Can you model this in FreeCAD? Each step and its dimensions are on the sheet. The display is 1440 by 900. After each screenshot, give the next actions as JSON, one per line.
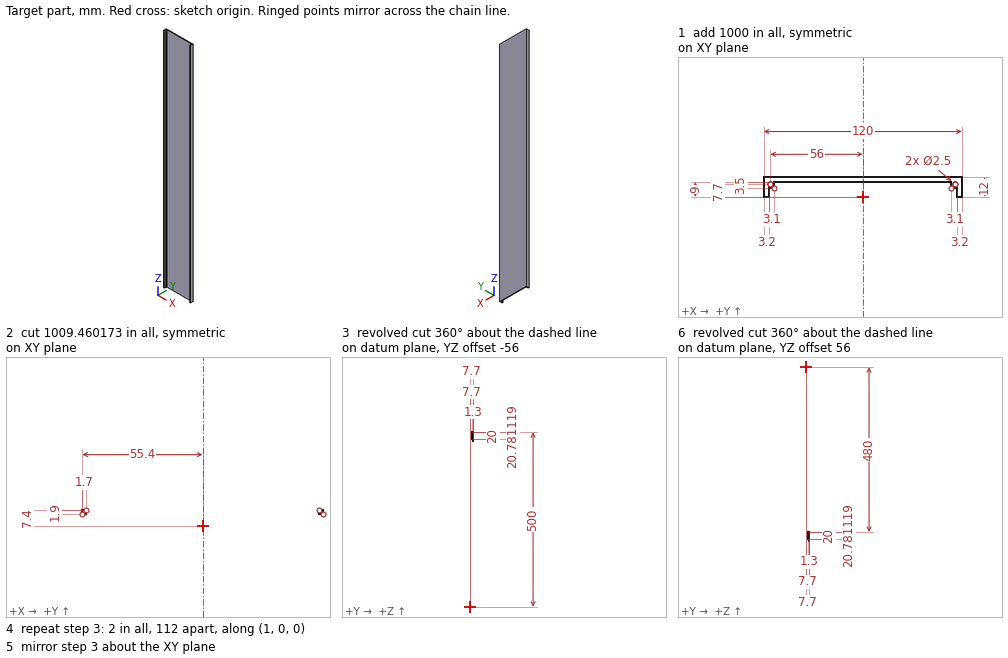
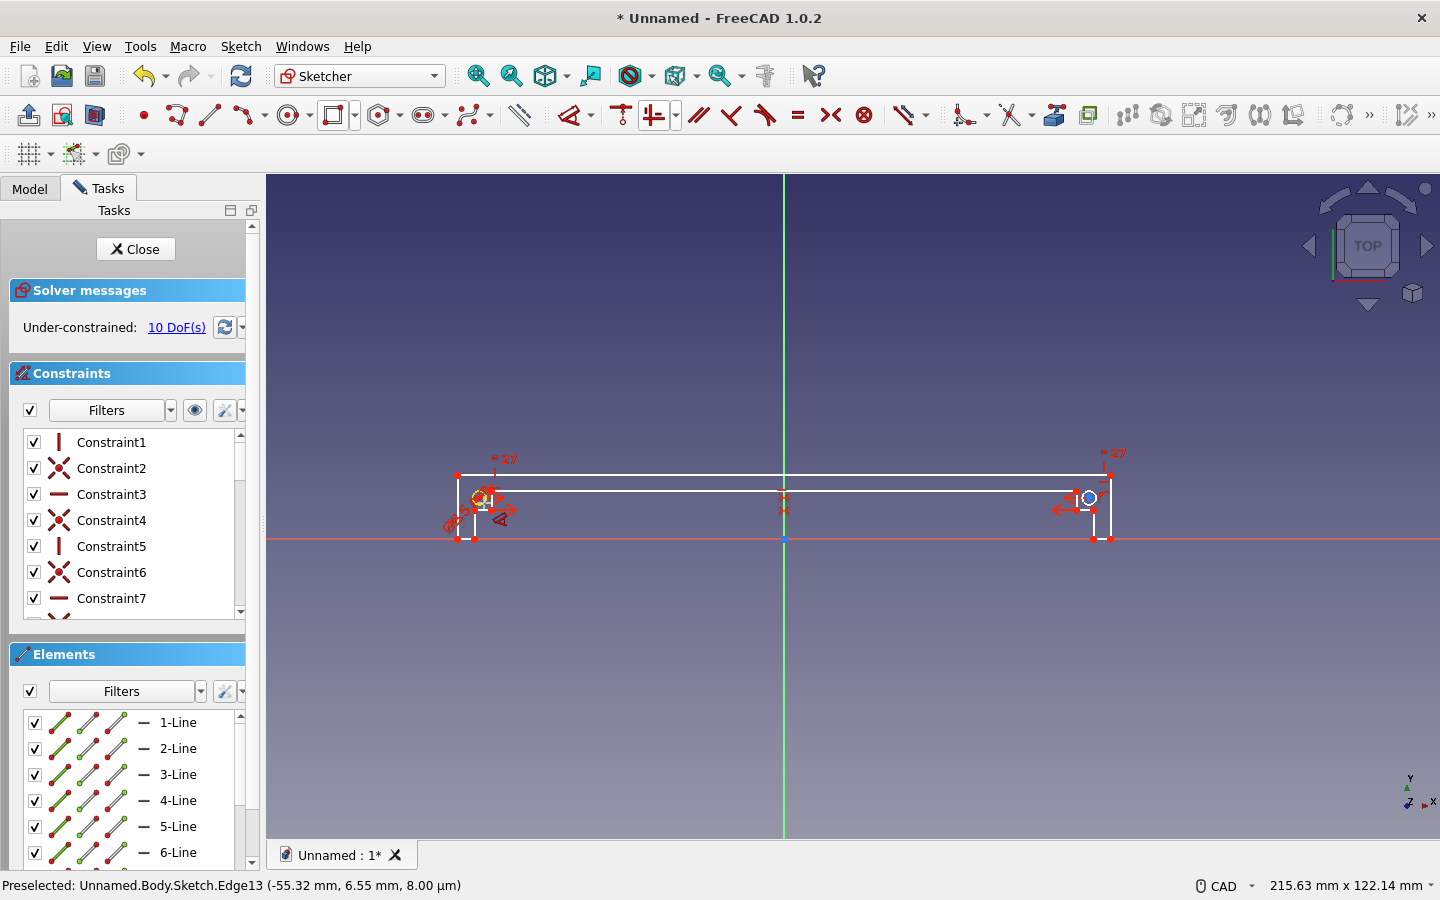
{"action": "left_click", "coordinate": [1111, 520]}
{"action": "left_click", "coordinate": [1145, 507]}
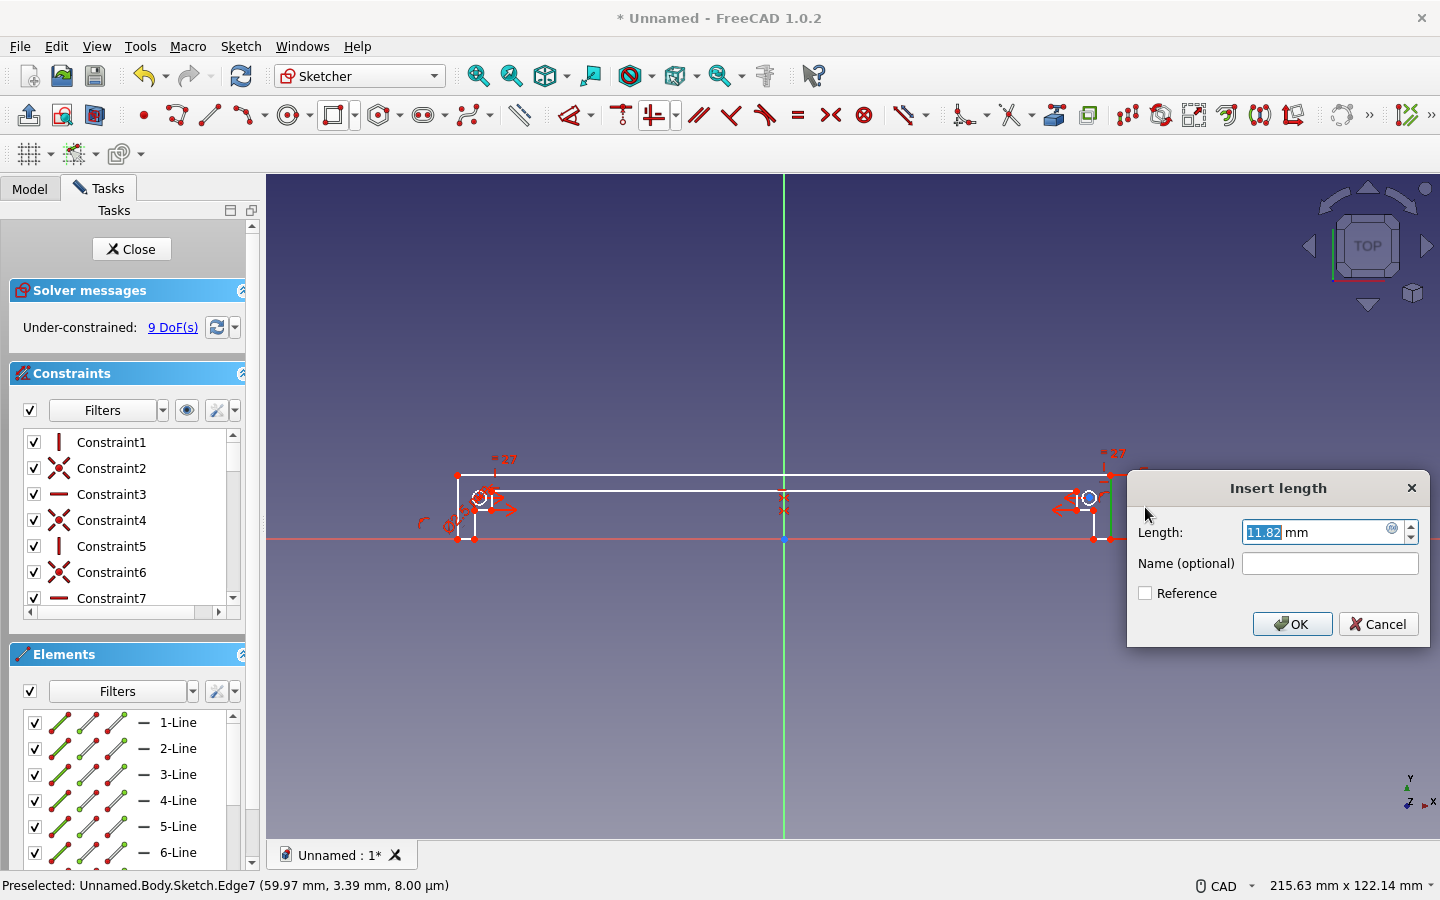
{"action": "type", "text": "12"}
{"action": "key", "text": "Return"}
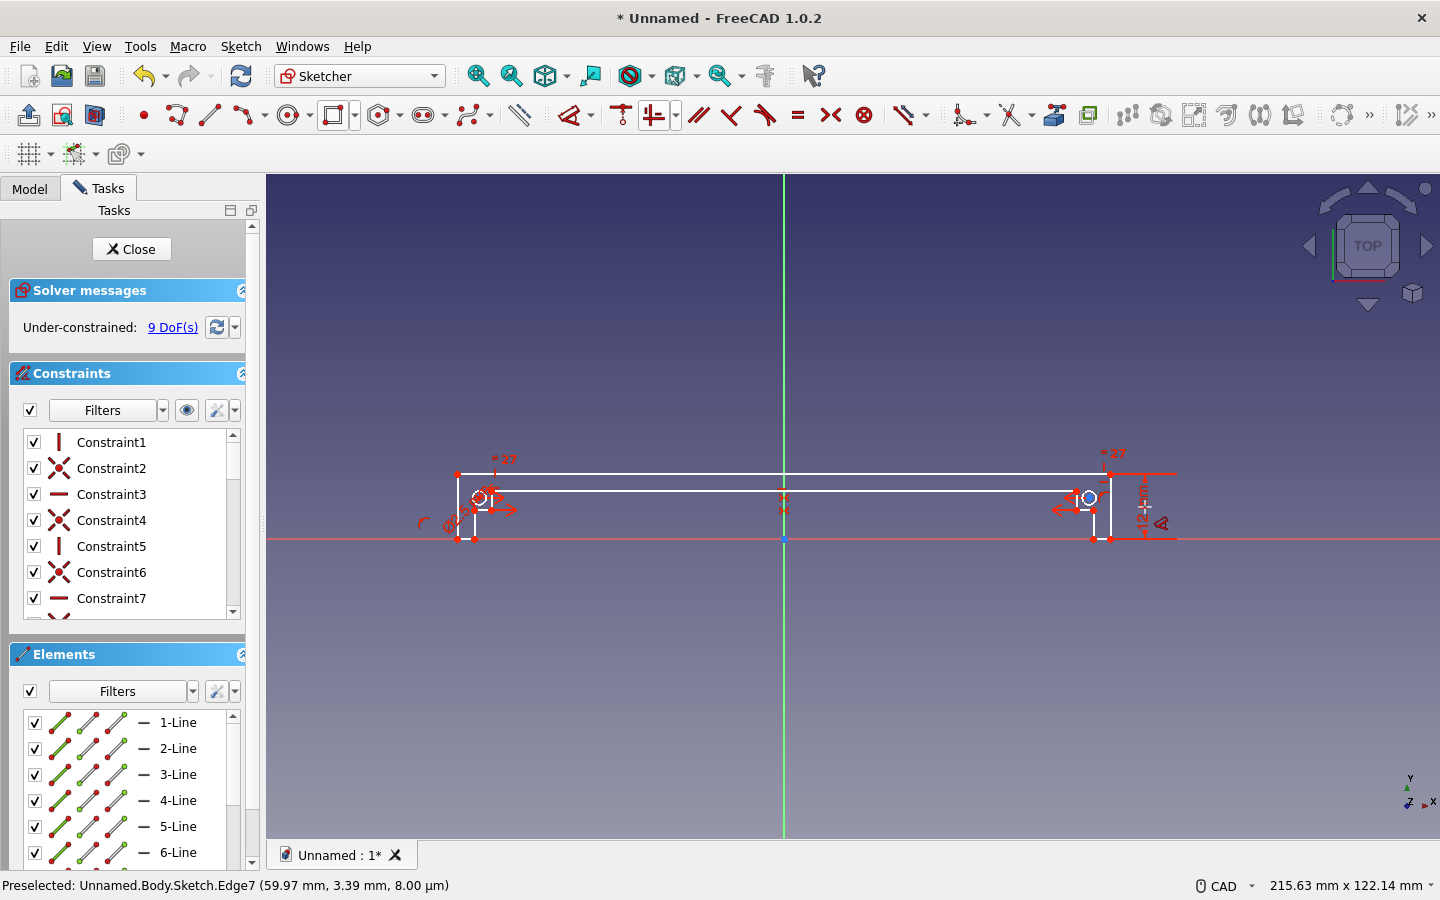
{"action": "left_click", "coordinate": [492, 491]}
{"action": "left_click", "coordinate": [818, 515]}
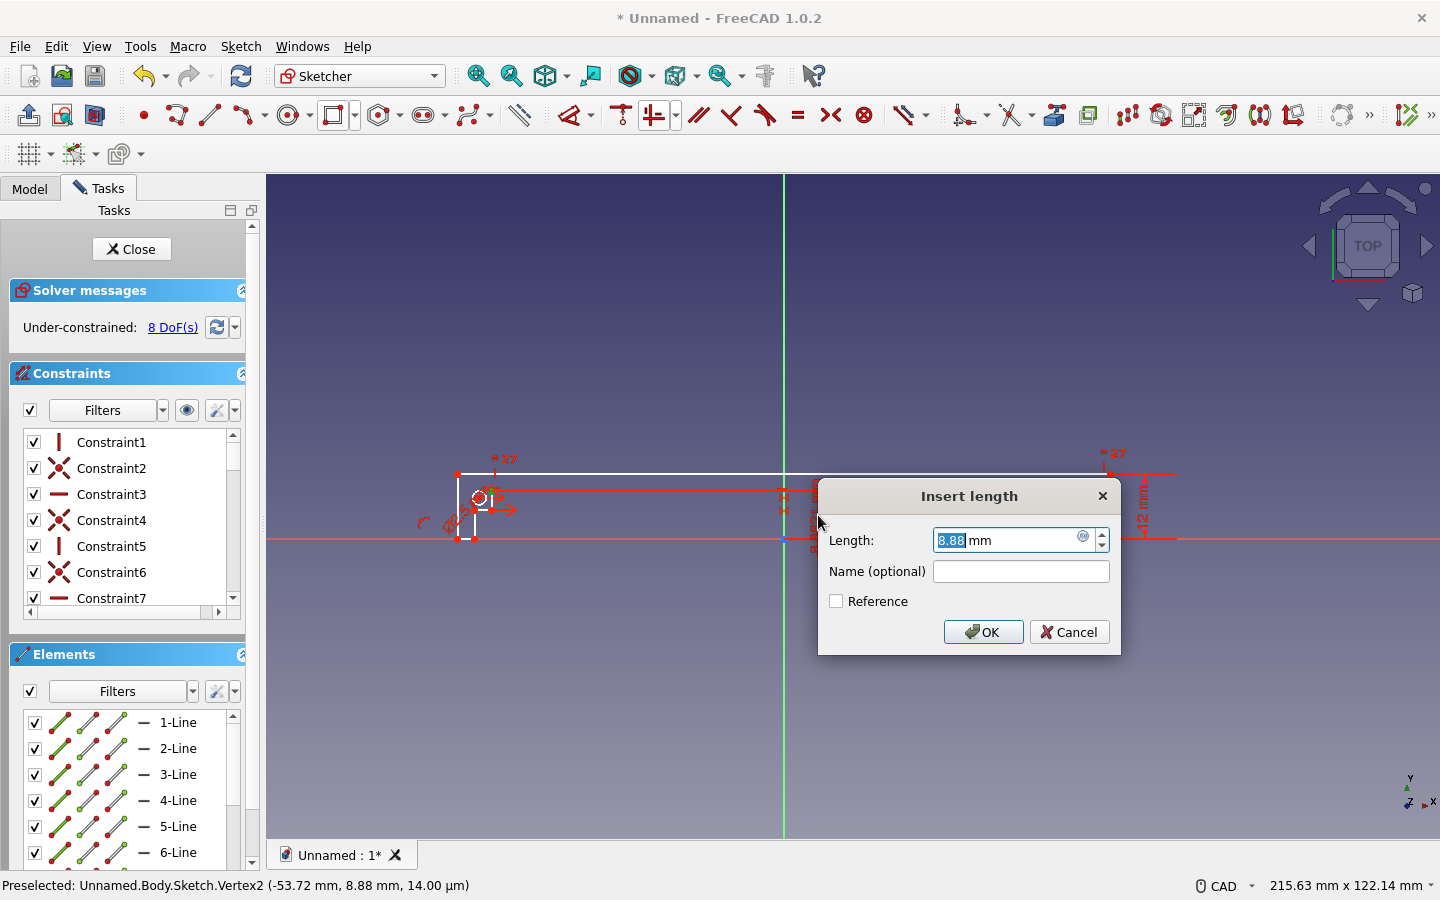
{"action": "type", "text": "9"}
{"action": "key", "text": "Return"}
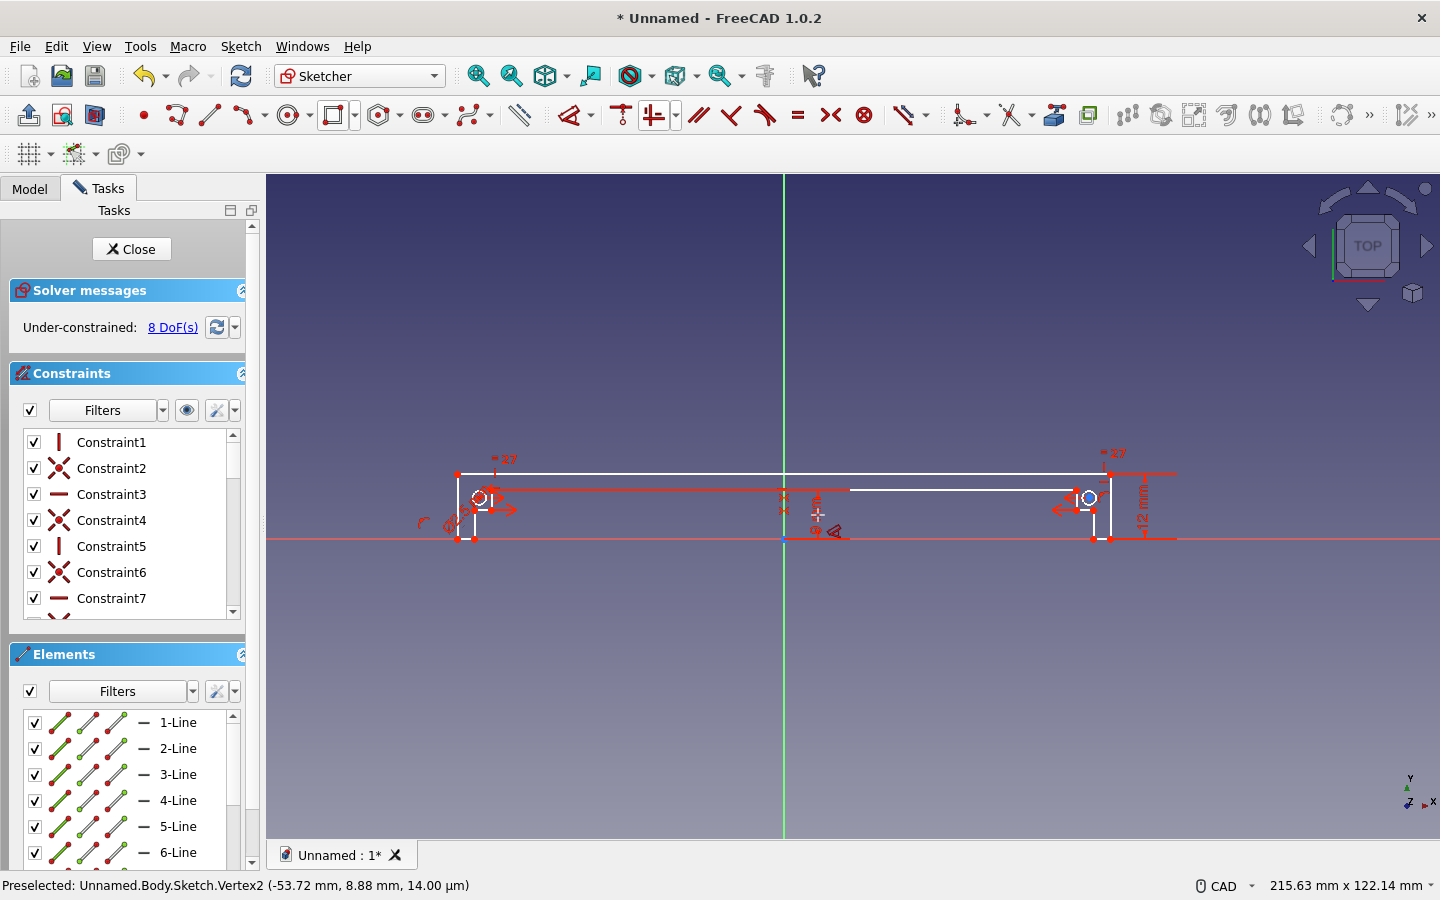
{"action": "left_click", "coordinate": [479, 498]}
{"action": "left_click", "coordinate": [632, 573]}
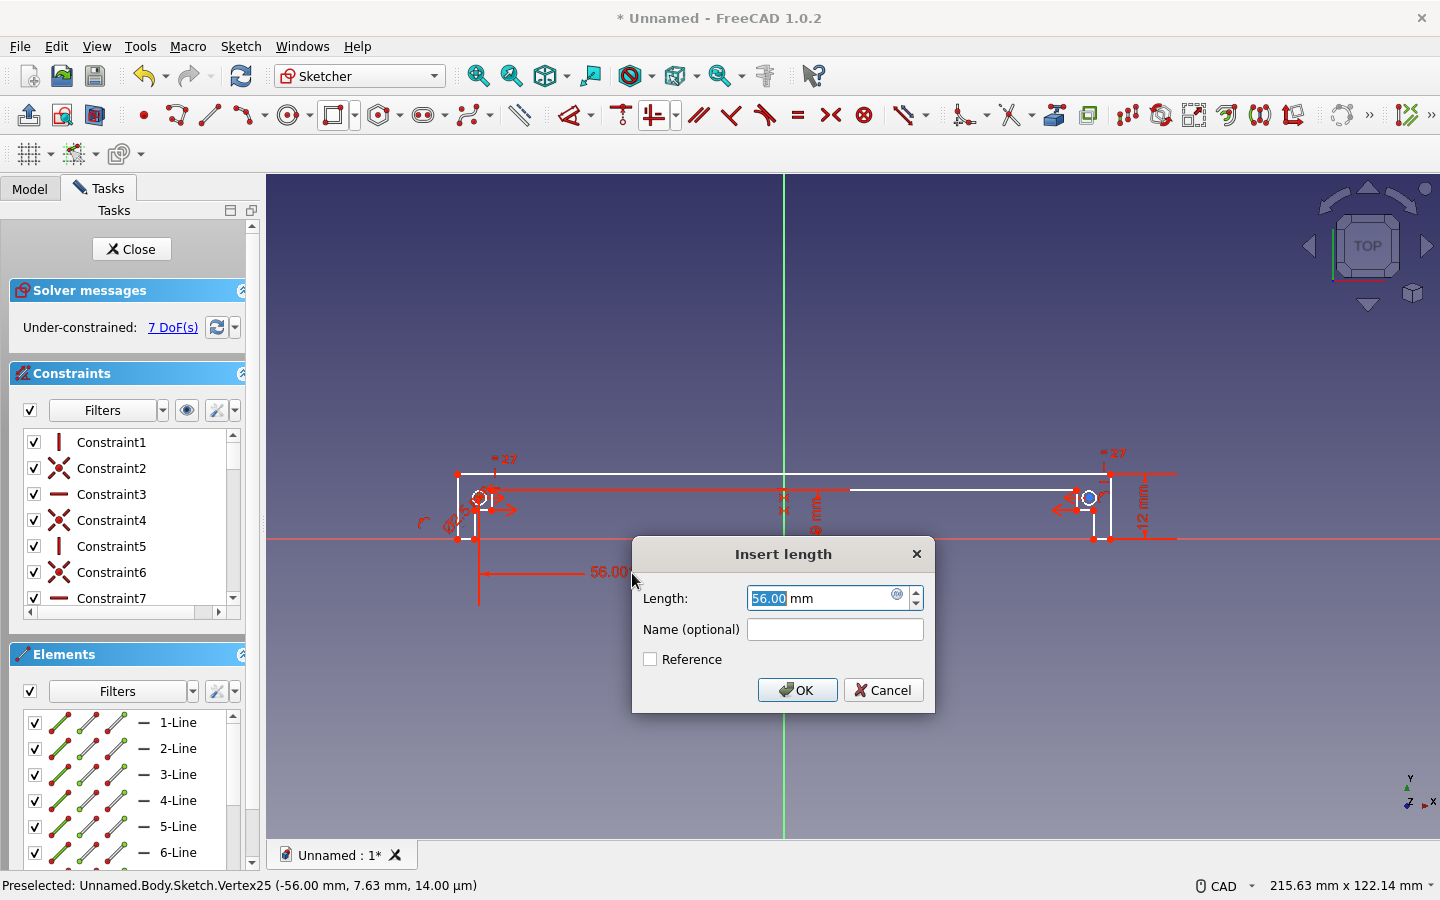
{"action": "type", "text": "56"}
{"action": "key", "text": "Return"}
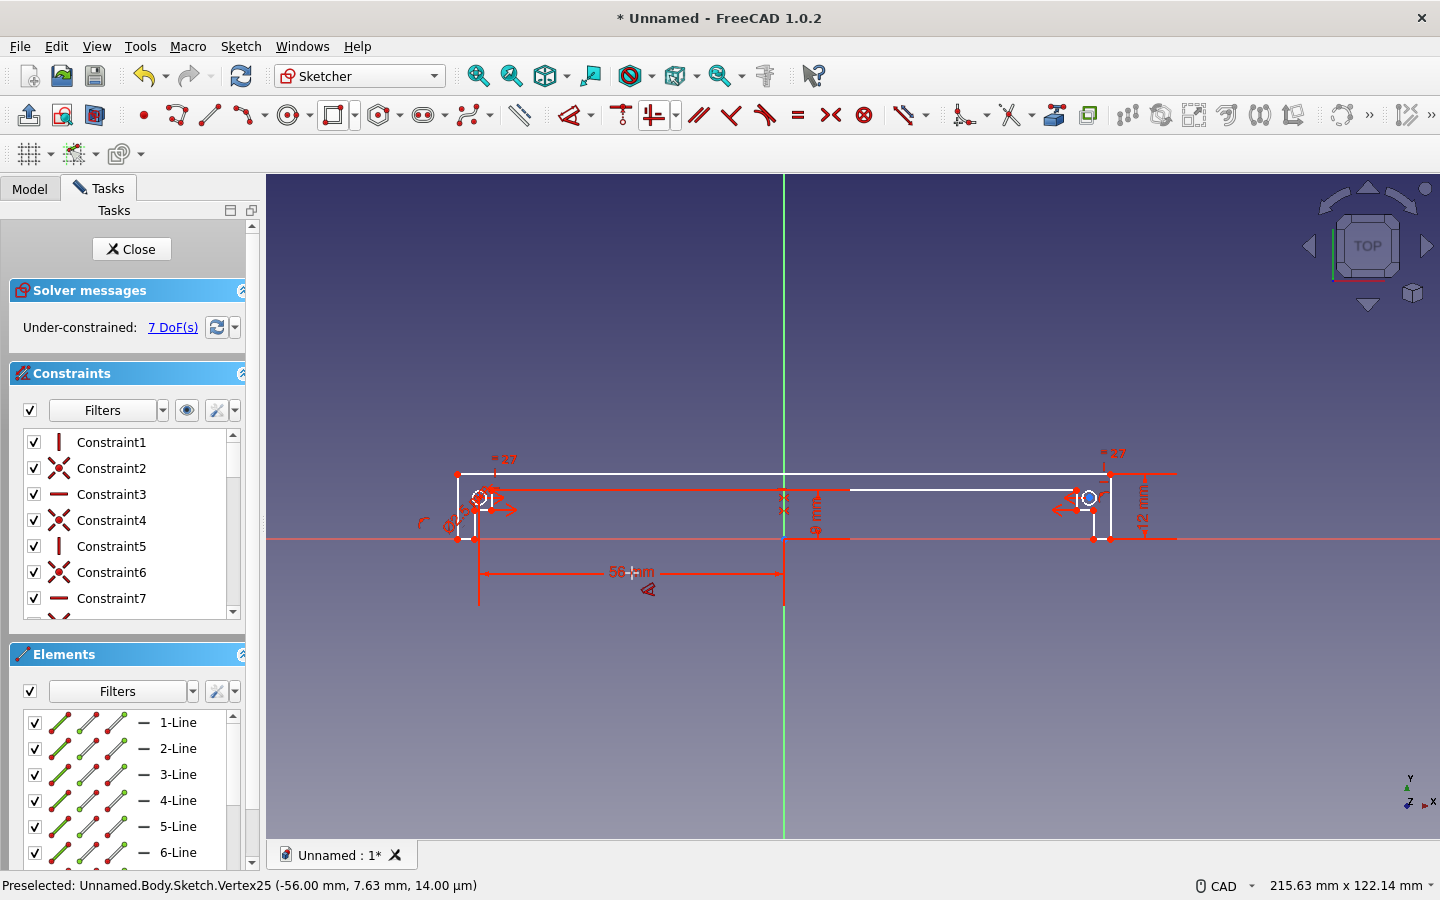
{"action": "scroll", "coordinate": [492, 502], "scroll_direction": "up", "scroll_amount": 4}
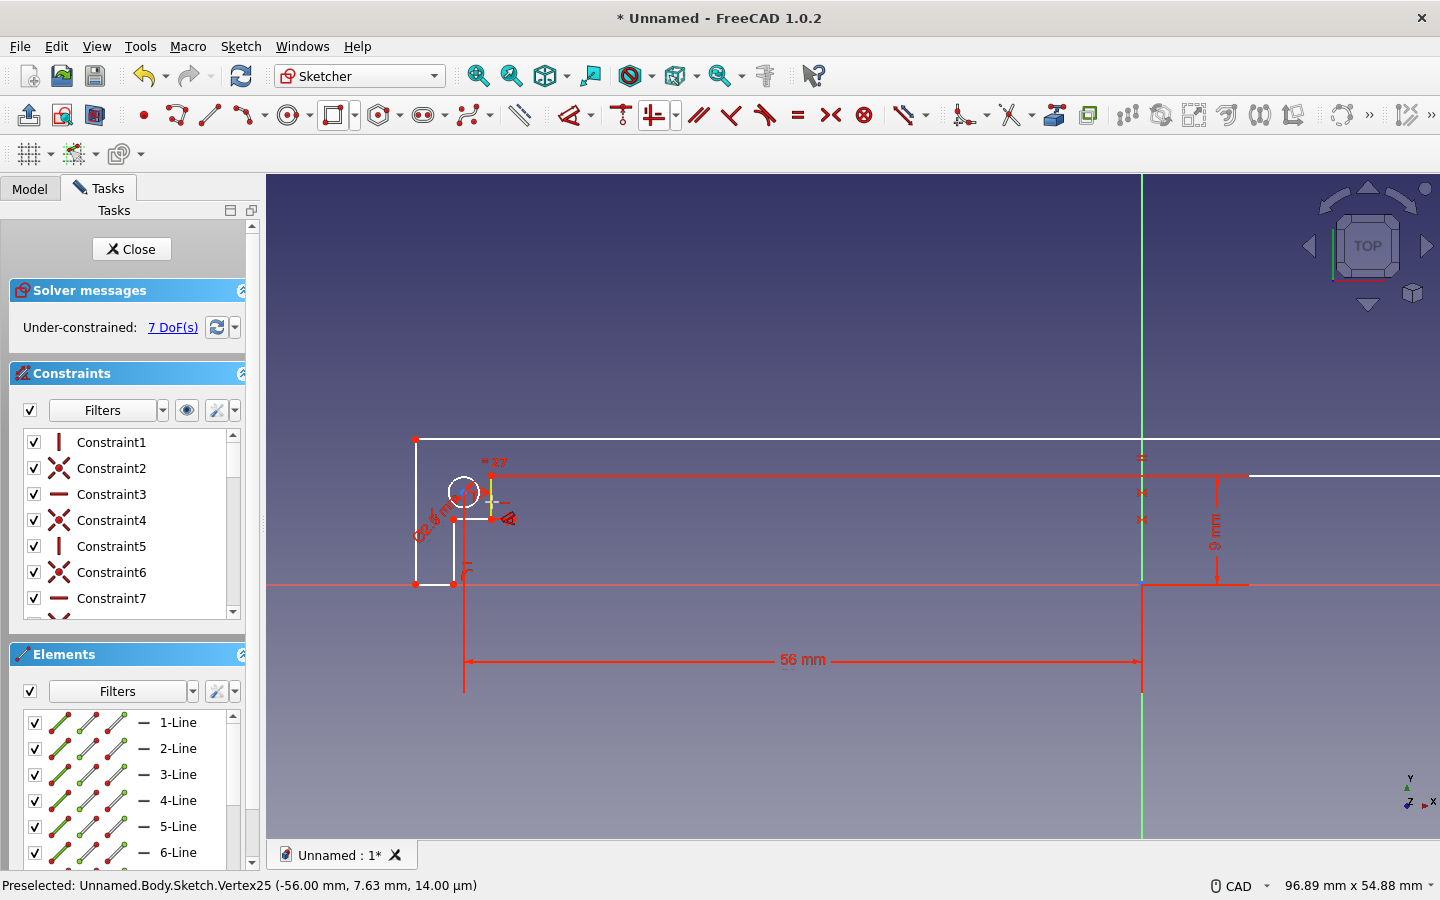
{"action": "left_click", "coordinate": [491, 502]}
{"action": "left_click", "coordinate": [525, 498]}